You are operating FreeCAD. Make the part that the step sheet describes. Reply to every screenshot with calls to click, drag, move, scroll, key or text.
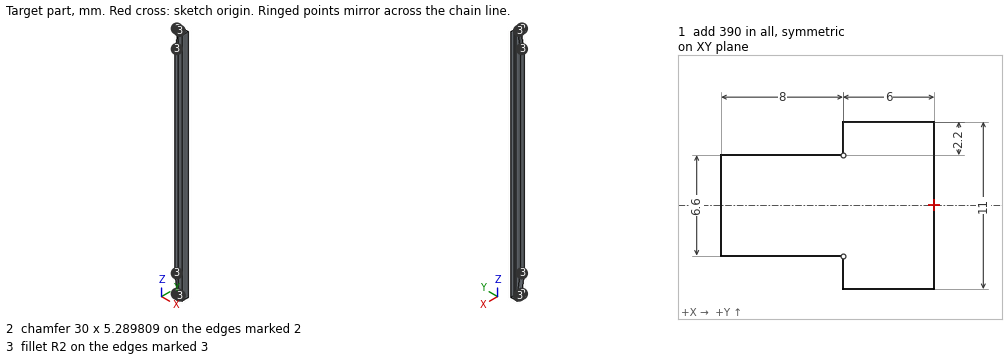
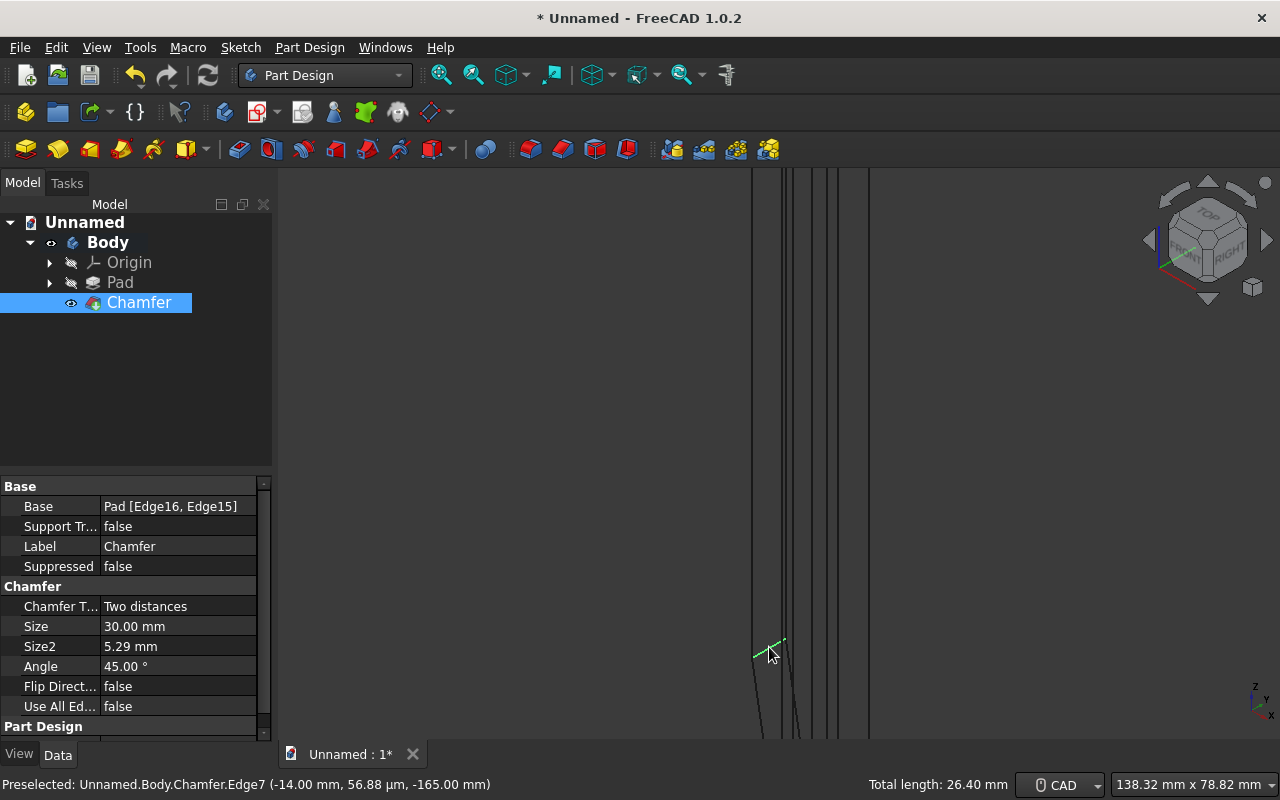
key(v)
key(1)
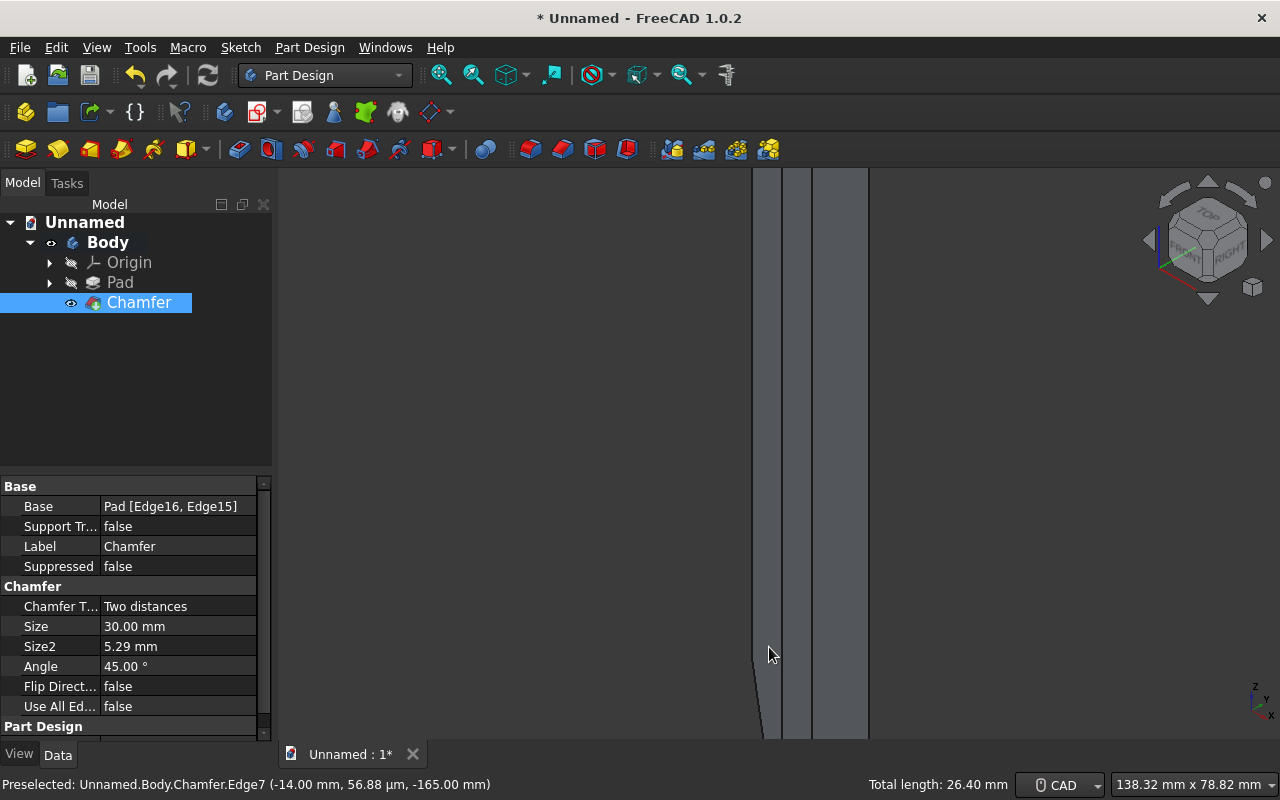
click(532, 150)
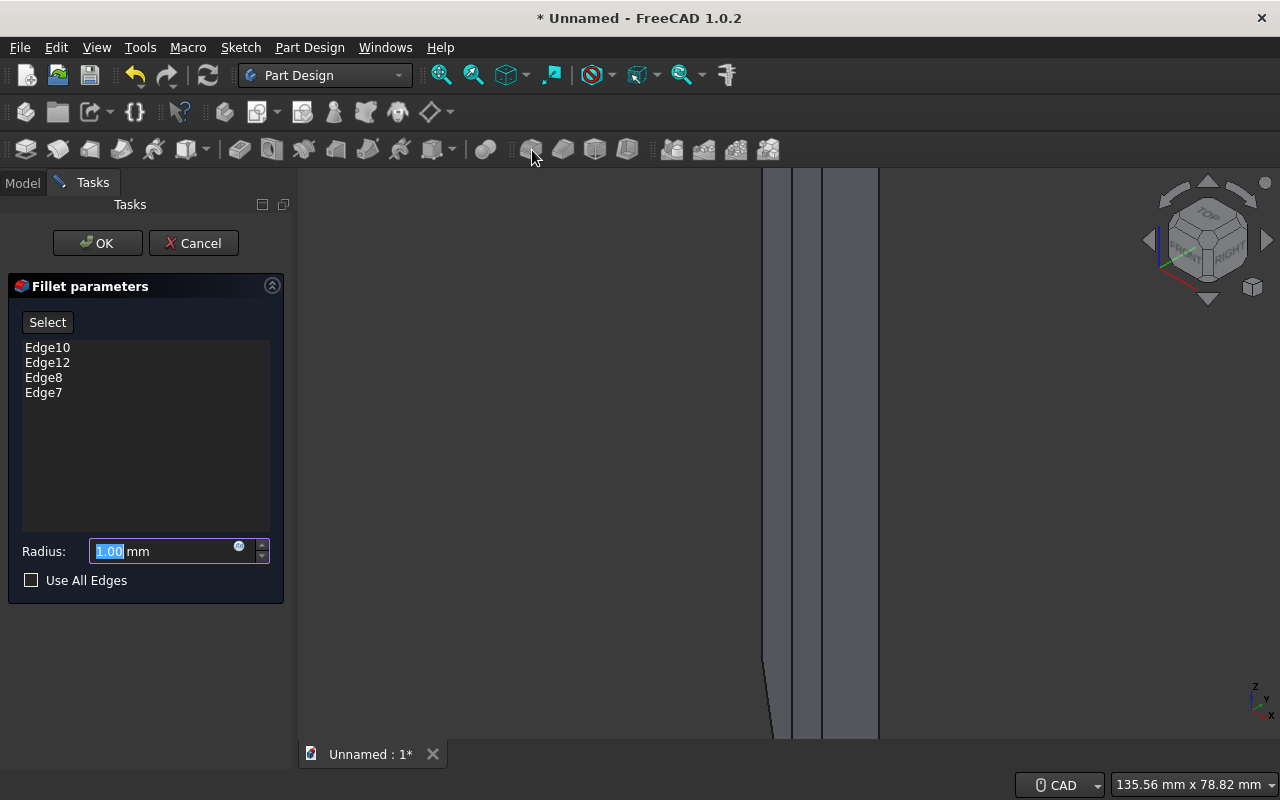
text(2)
key(Tab)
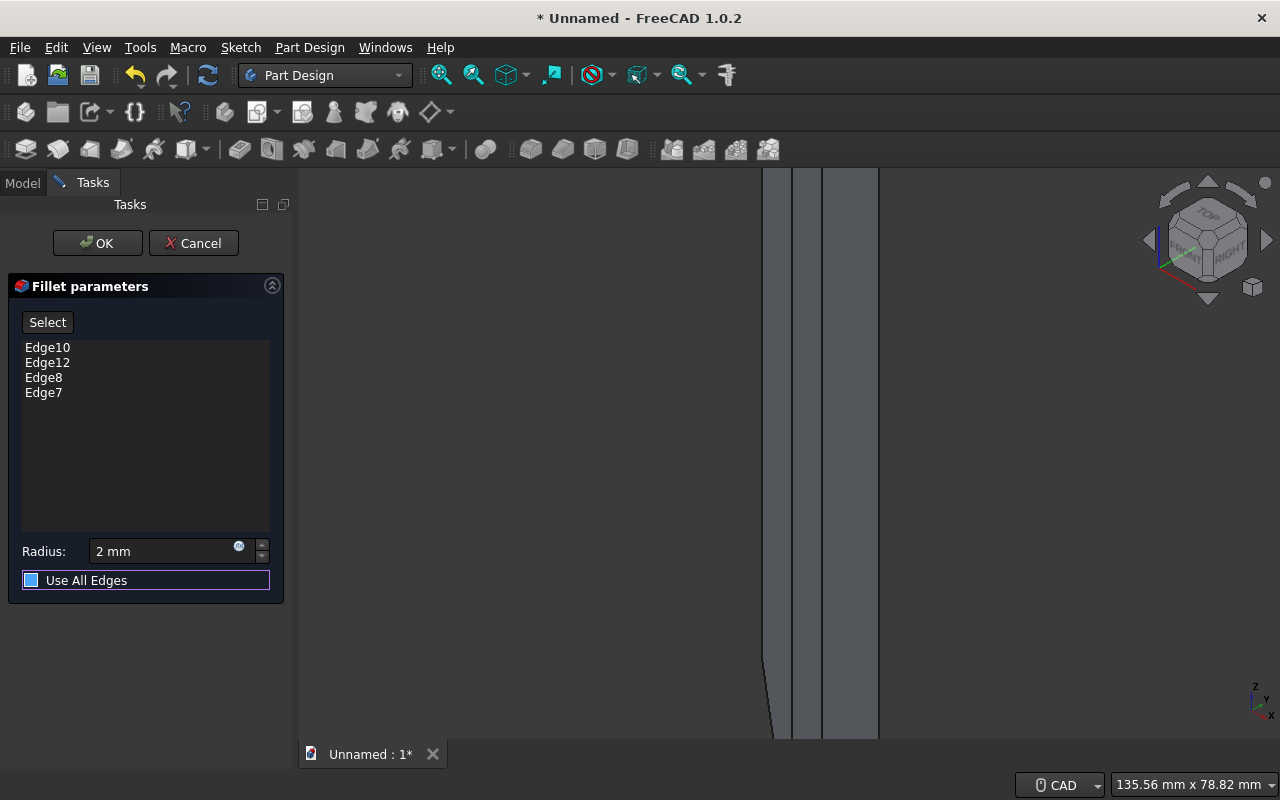
click(98, 243)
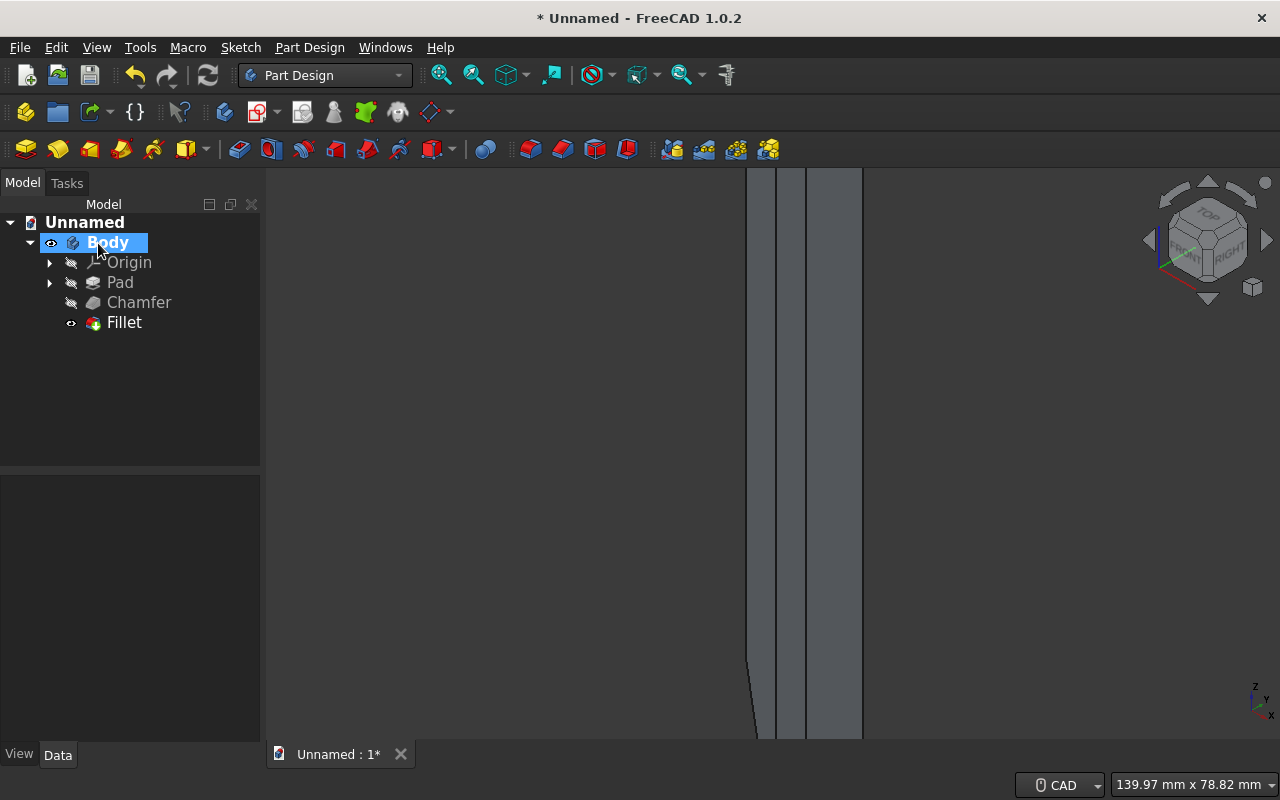
click(442, 76)